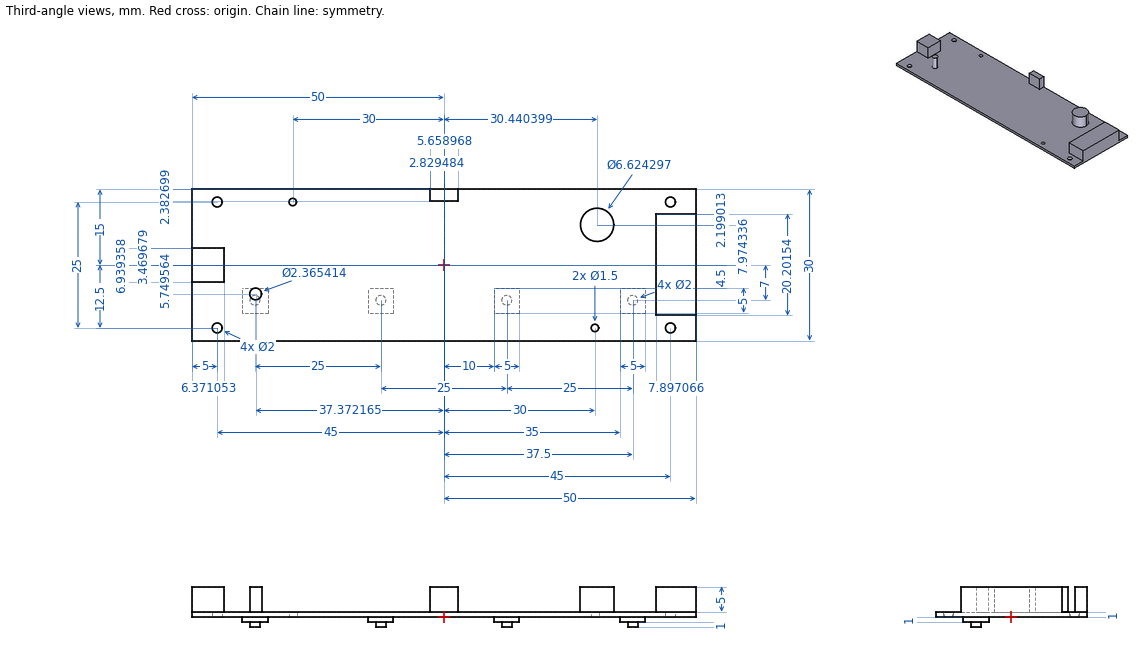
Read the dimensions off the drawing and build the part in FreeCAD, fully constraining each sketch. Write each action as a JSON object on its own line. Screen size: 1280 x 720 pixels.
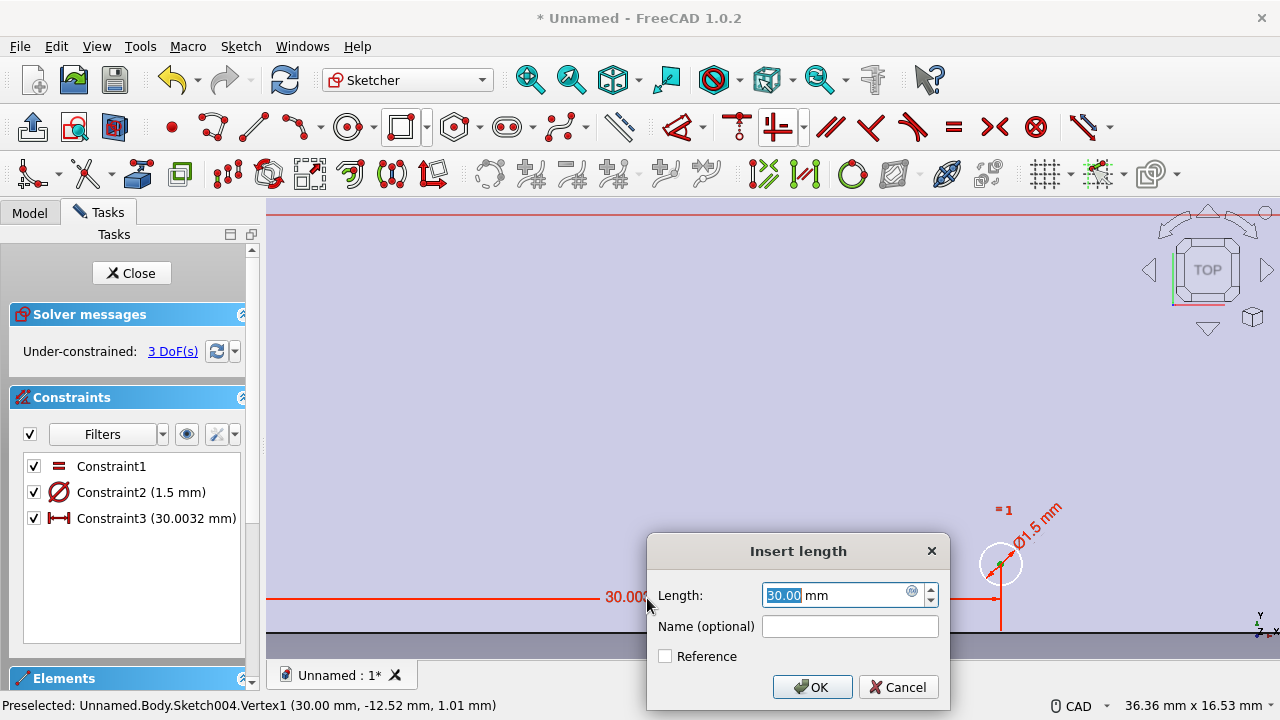
{"action": "type", "text": "30"}
{"action": "key", "text": "Return"}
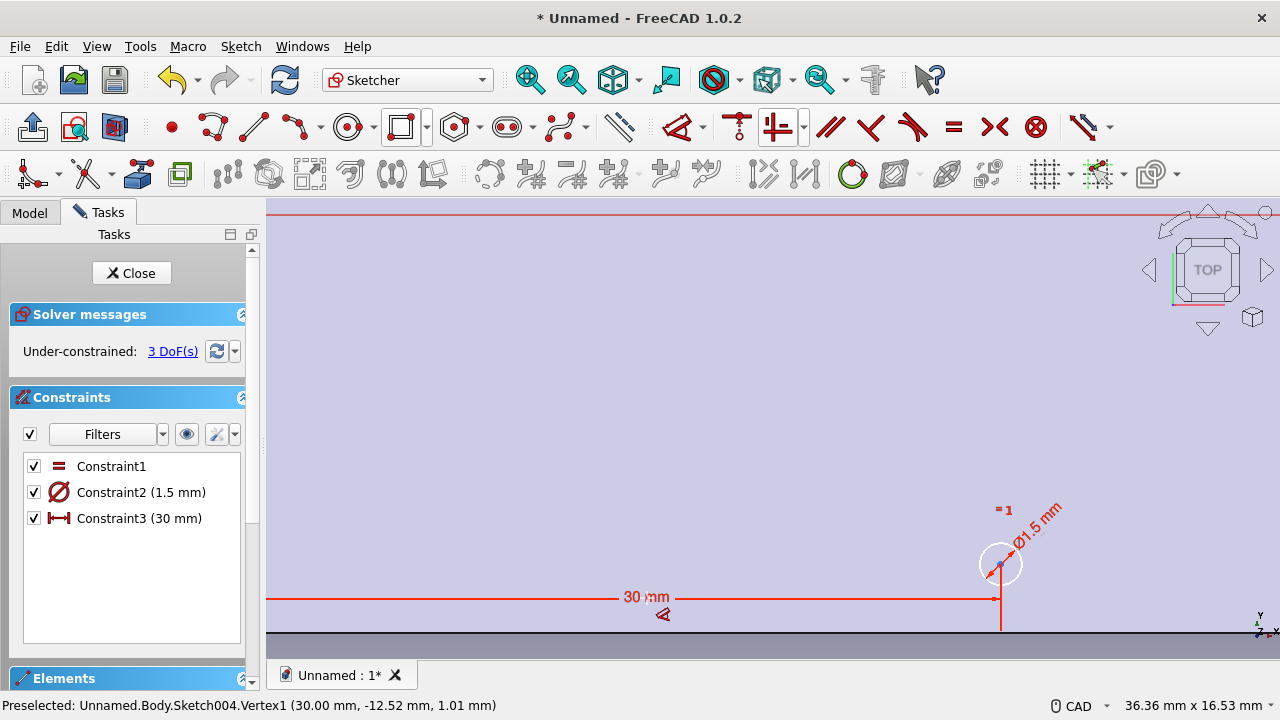
{"action": "scroll", "coordinate": [1019, 553], "scroll_direction": "down", "scroll_amount": 5}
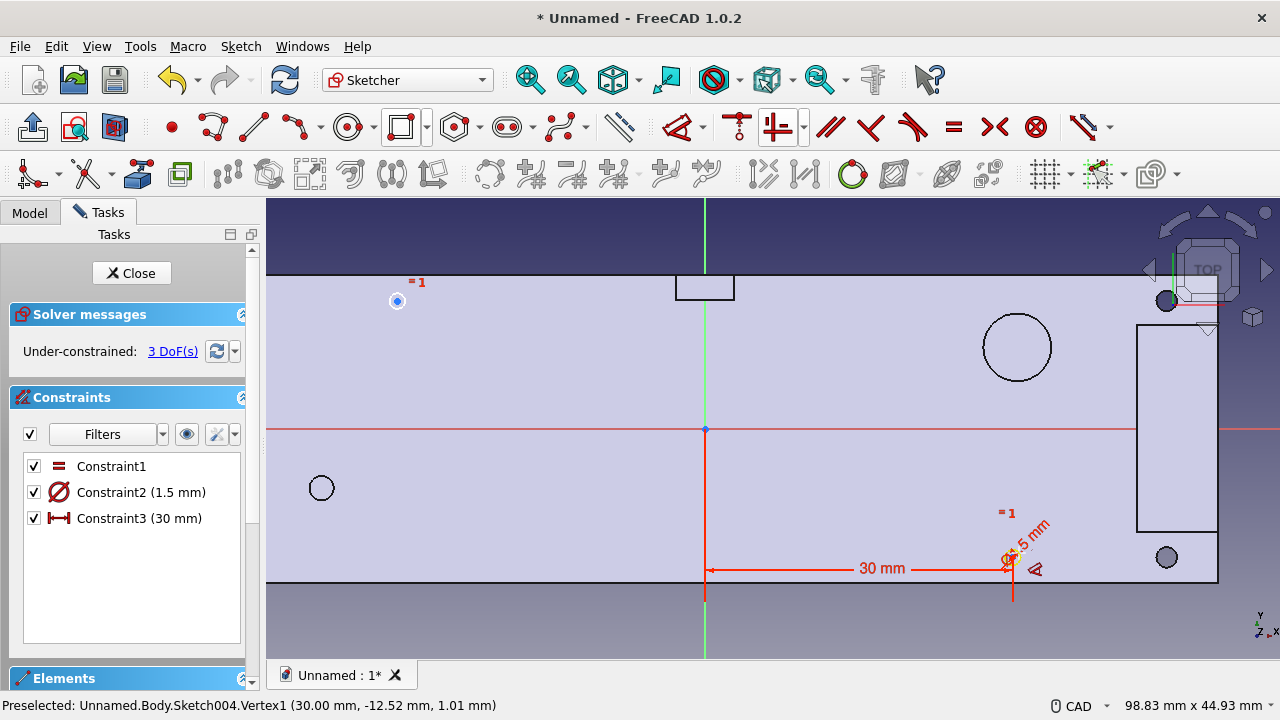
{"action": "left_click", "coordinate": [397, 301]}
{"action": "left_click", "coordinate": [551, 267]}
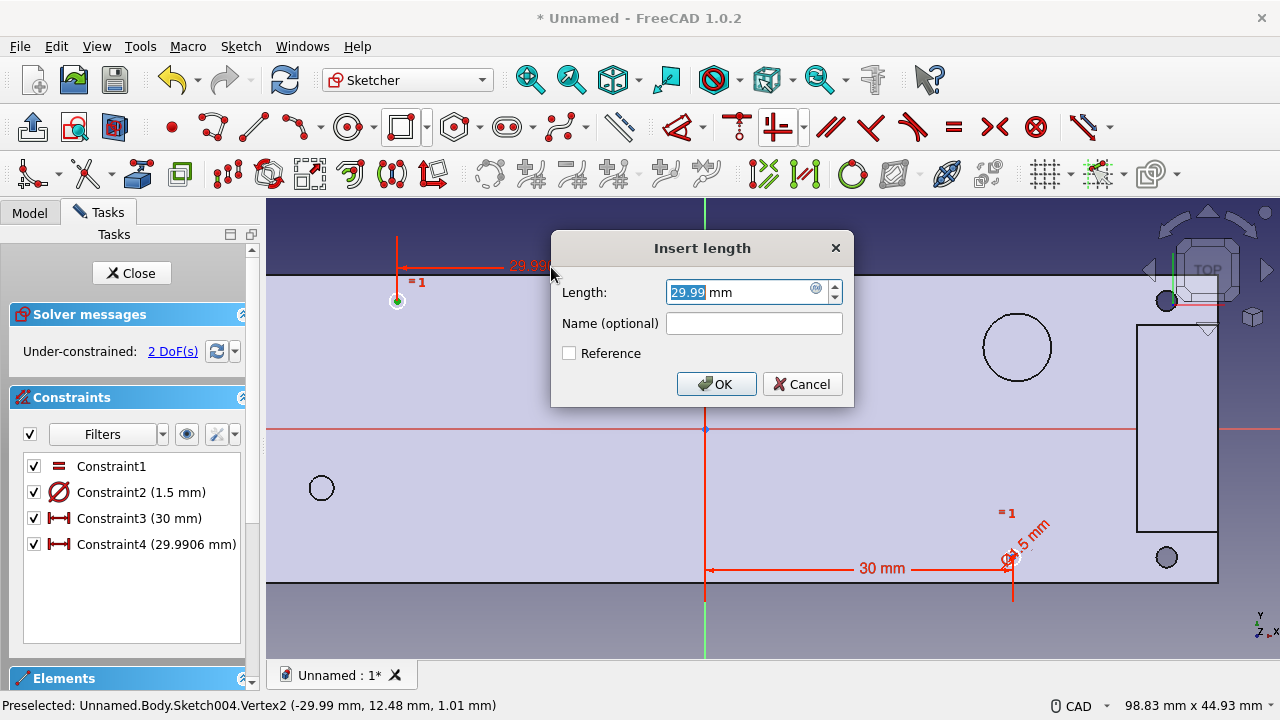
{"action": "type", "text": "30"}
{"action": "key", "text": "Return"}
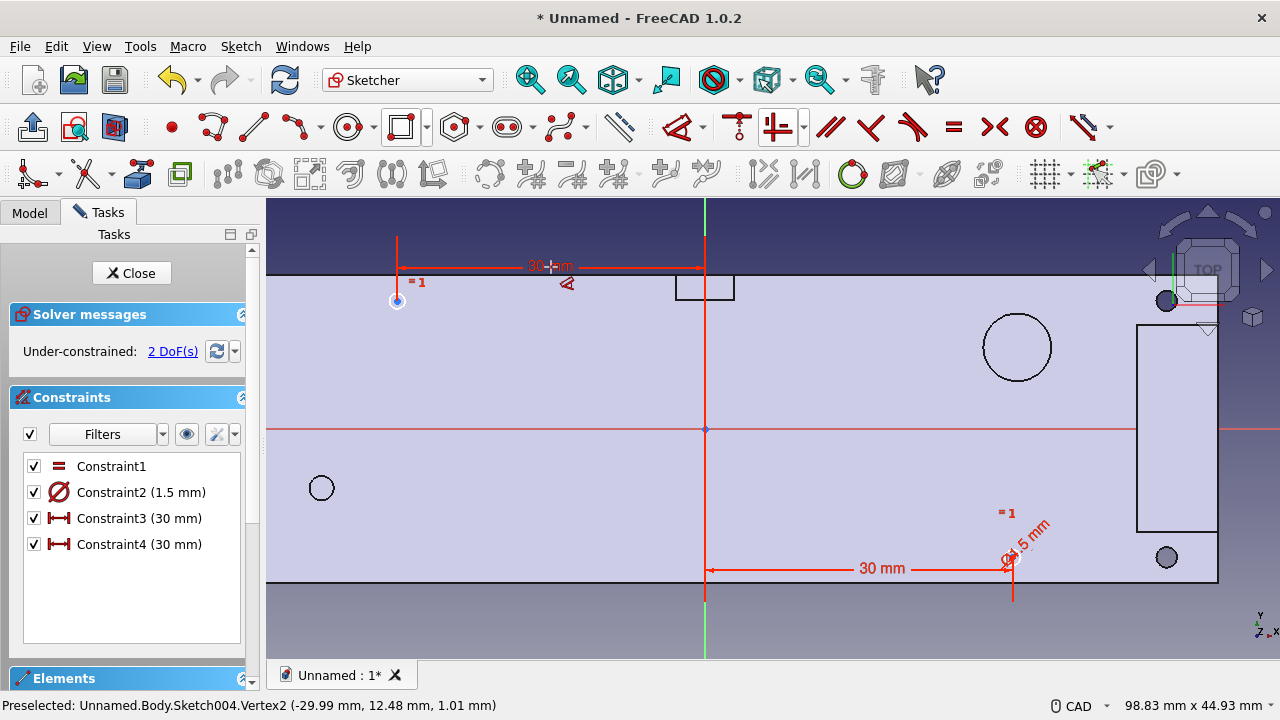
{"action": "left_click", "coordinate": [1013, 558]}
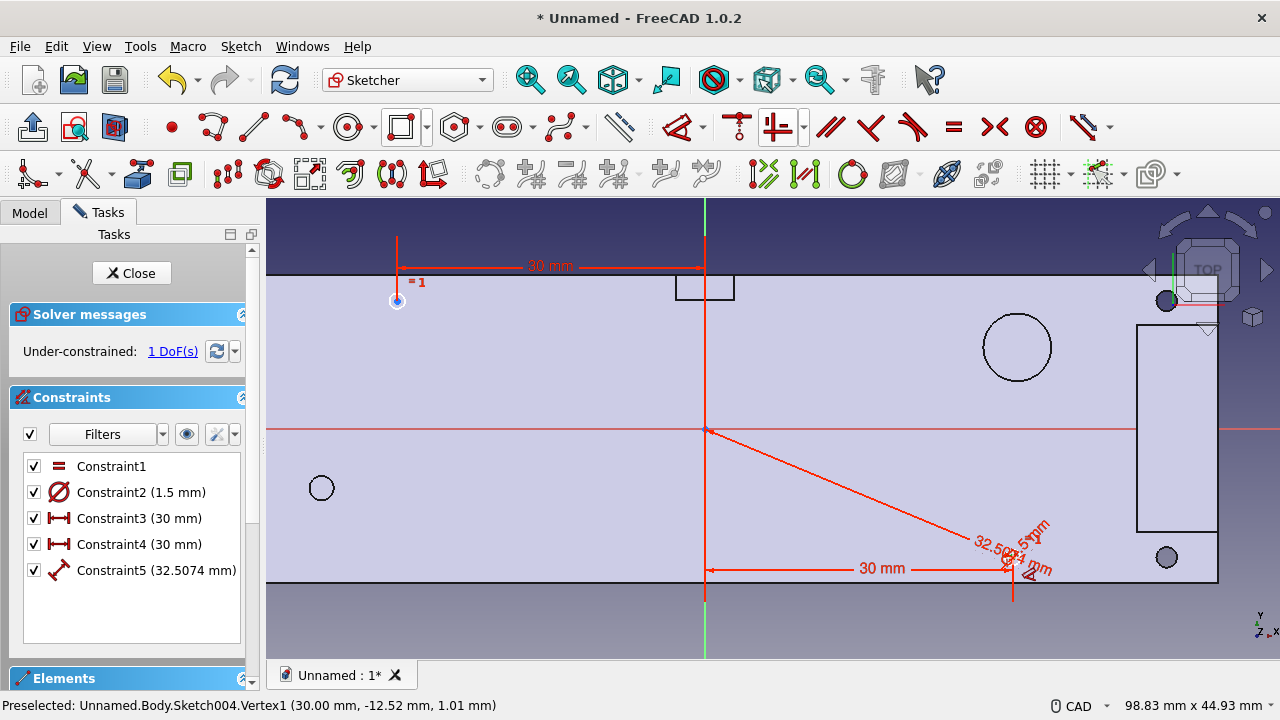
{"action": "left_click", "coordinate": [397, 301]}
{"action": "left_click", "coordinate": [1047, 370]}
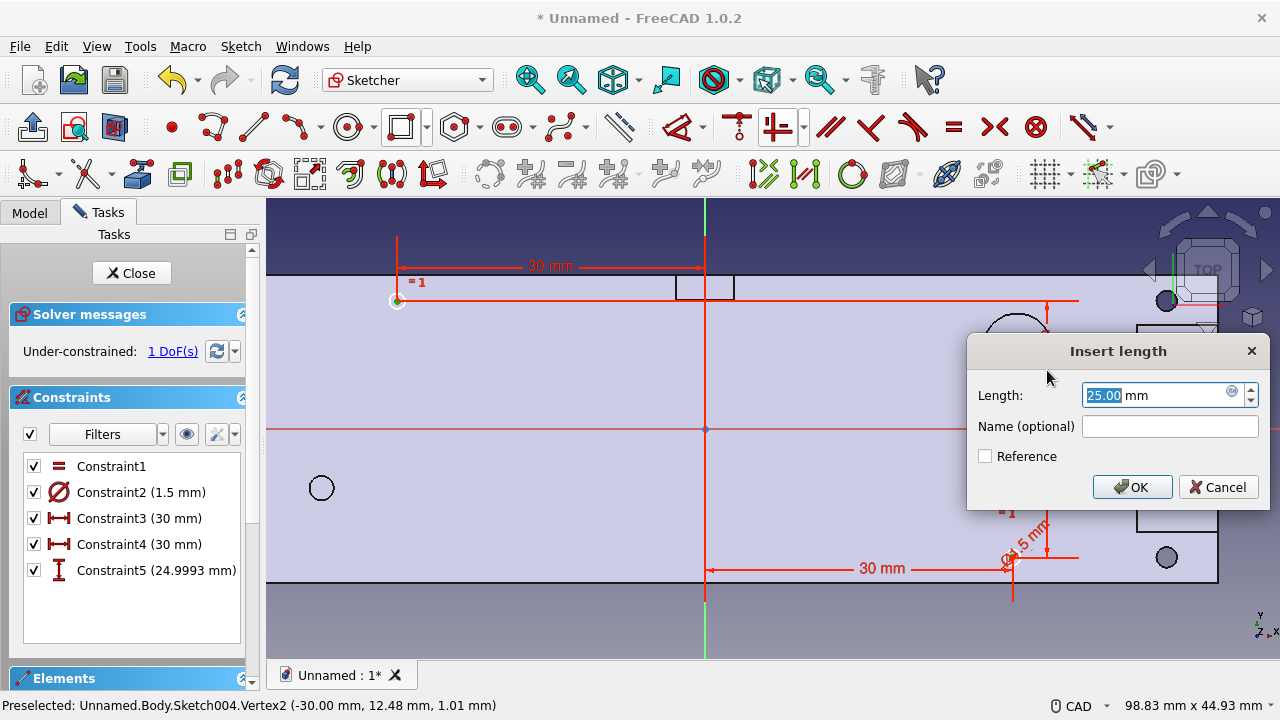
{"action": "type", "text": "25"}
{"action": "key", "text": "Return"}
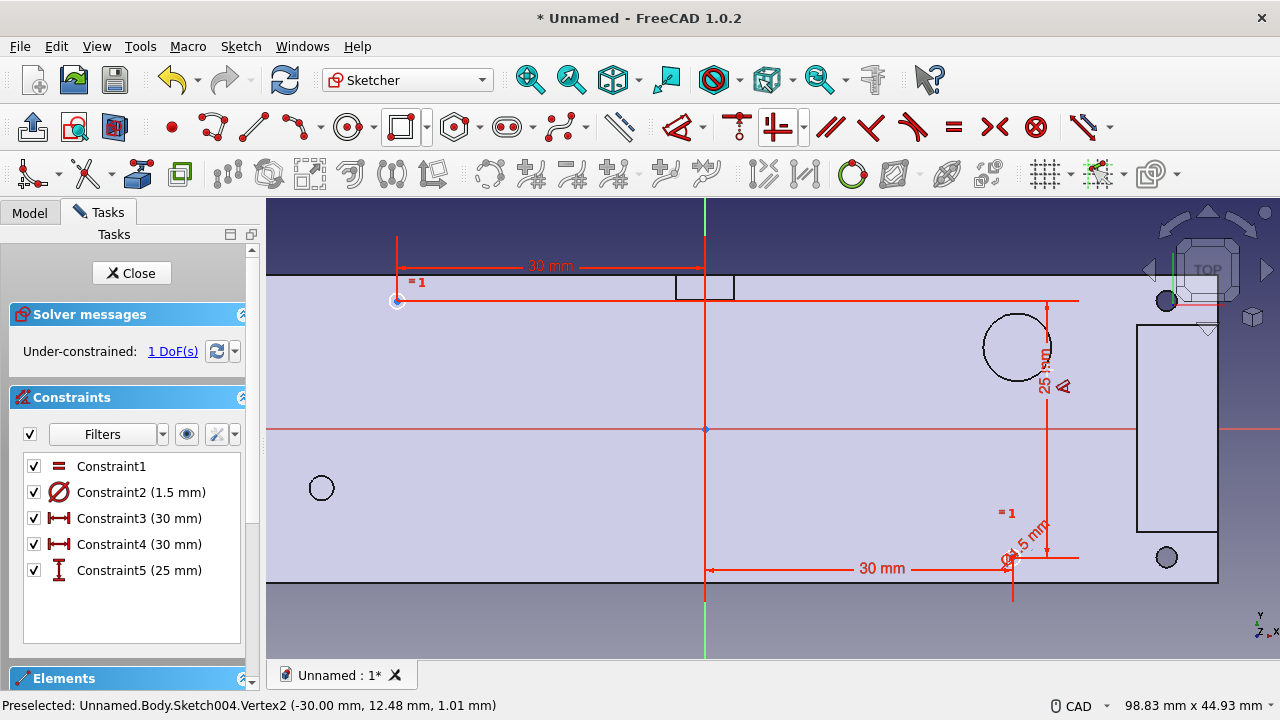
{"action": "left_click", "coordinate": [1013, 558]}
{"action": "left_click", "coordinate": [1047, 493]}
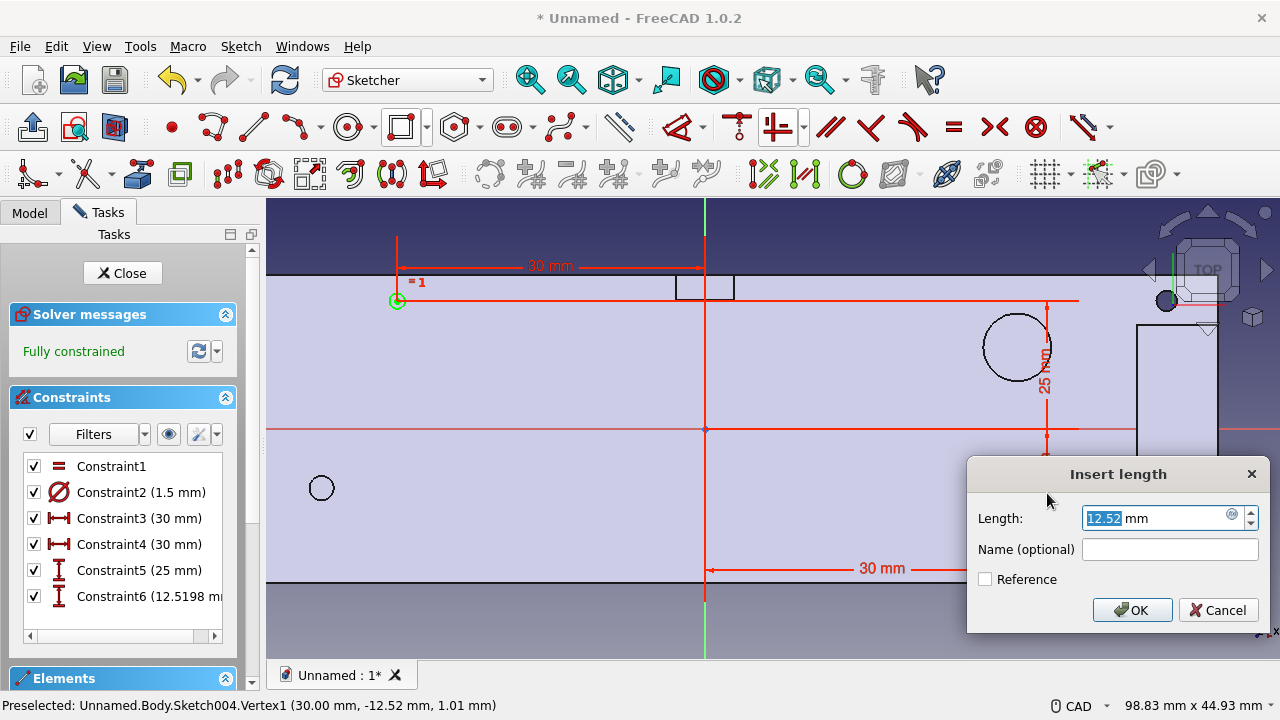
{"action": "type", "text": "12.5"}
{"action": "key", "text": "Return"}
{"action": "key", "text": "Escape"}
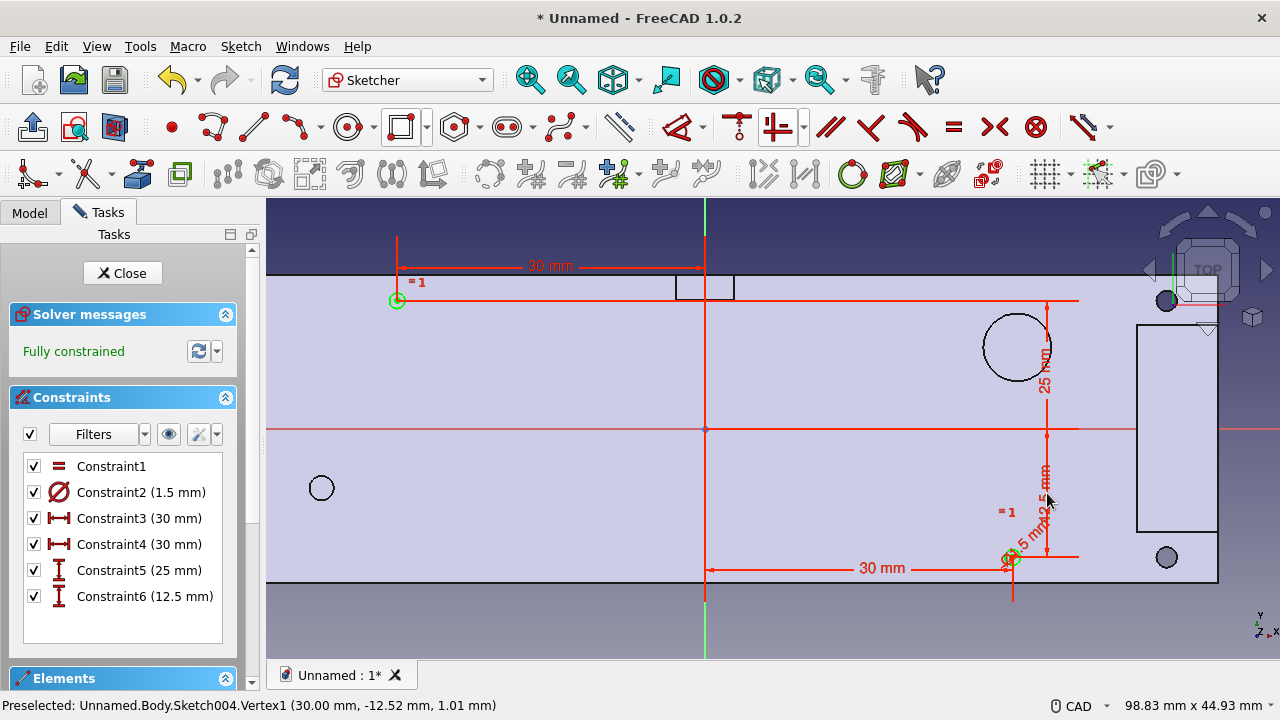
{"action": "left_click", "coordinate": [123, 273]}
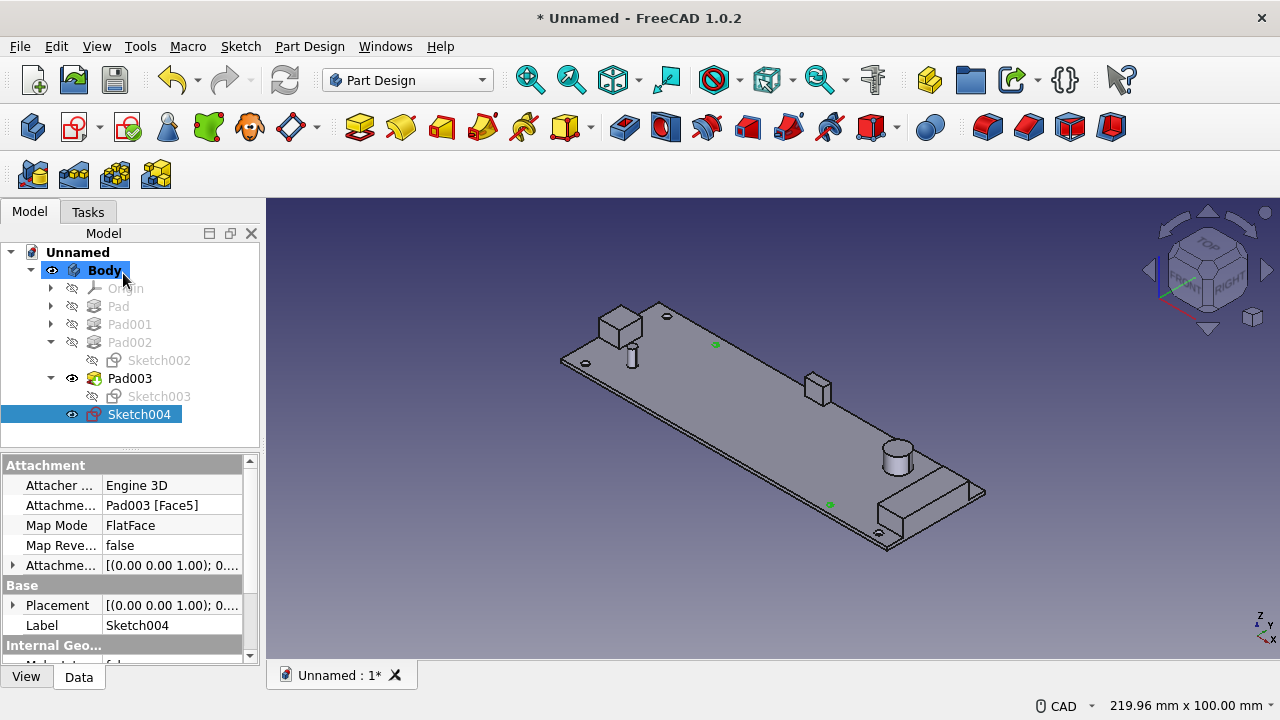
{"action": "left_click", "coordinate": [625, 128]}